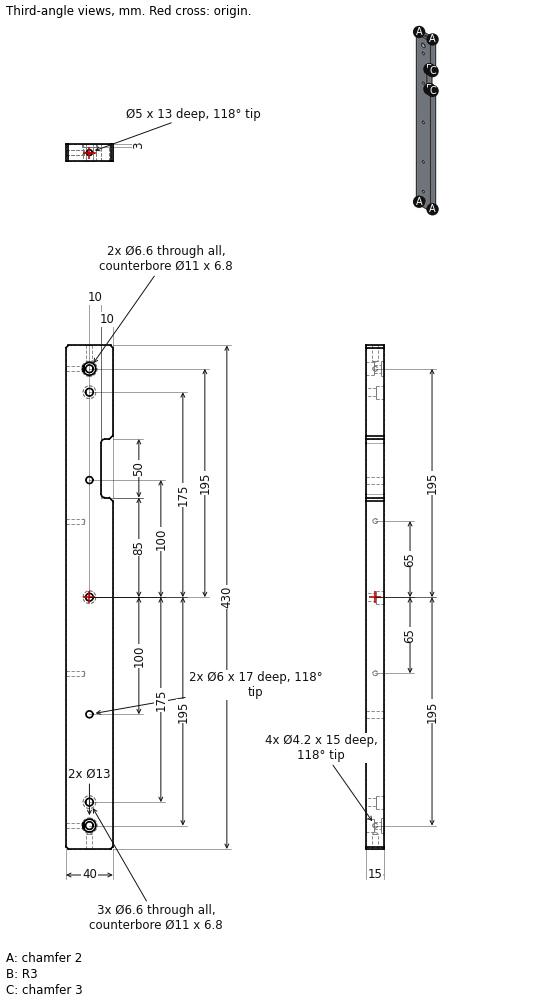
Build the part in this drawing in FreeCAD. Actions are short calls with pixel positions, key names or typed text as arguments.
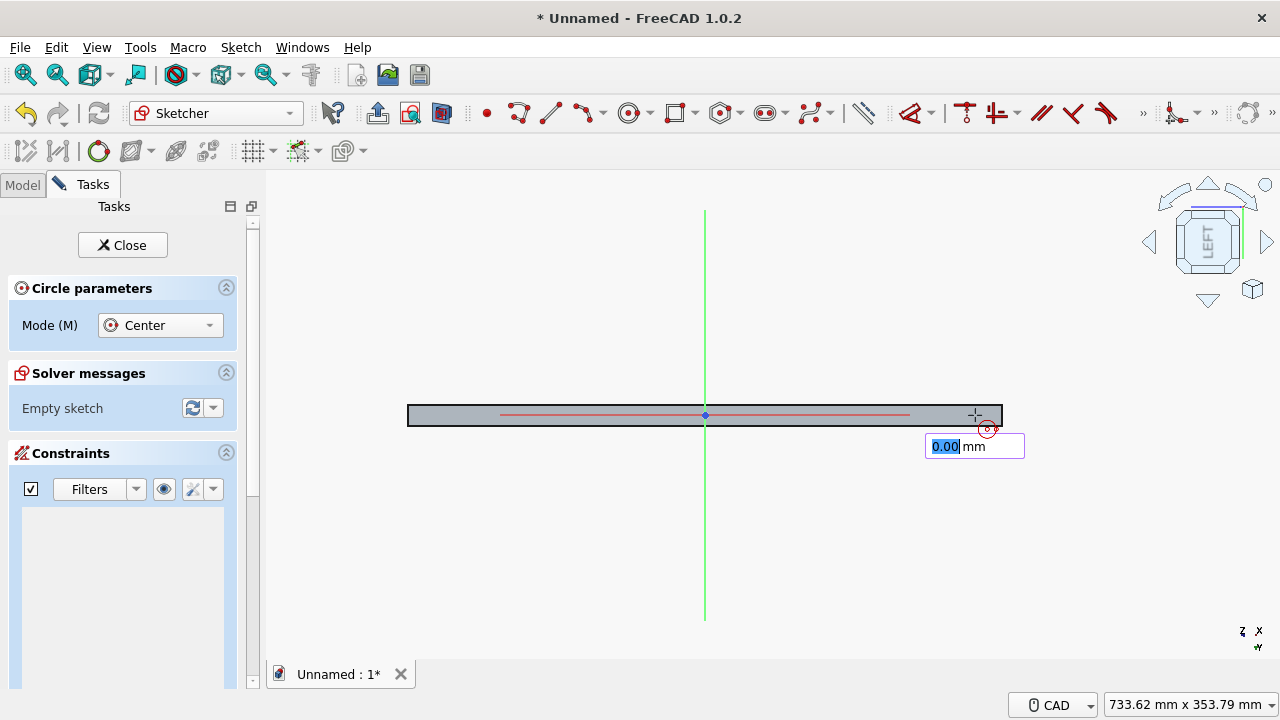
scroll(976, 412, up, 9)
move(971, 412)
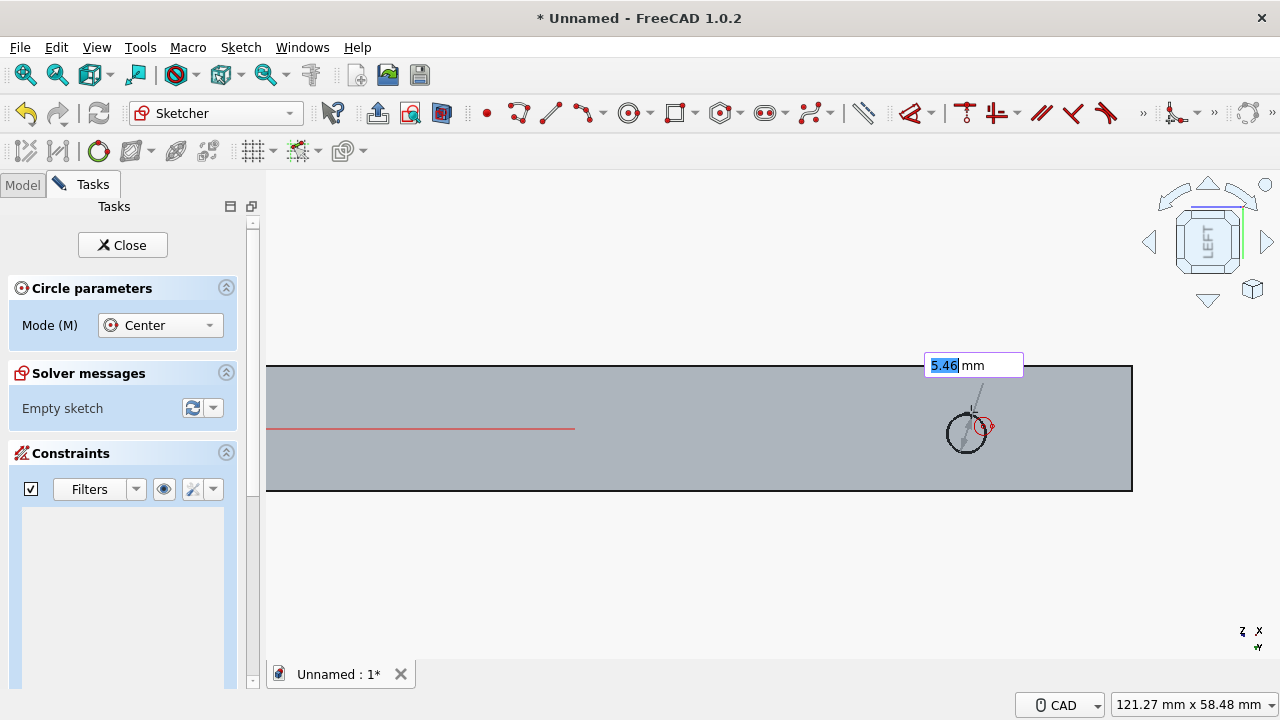
text(4.2)
key(Return)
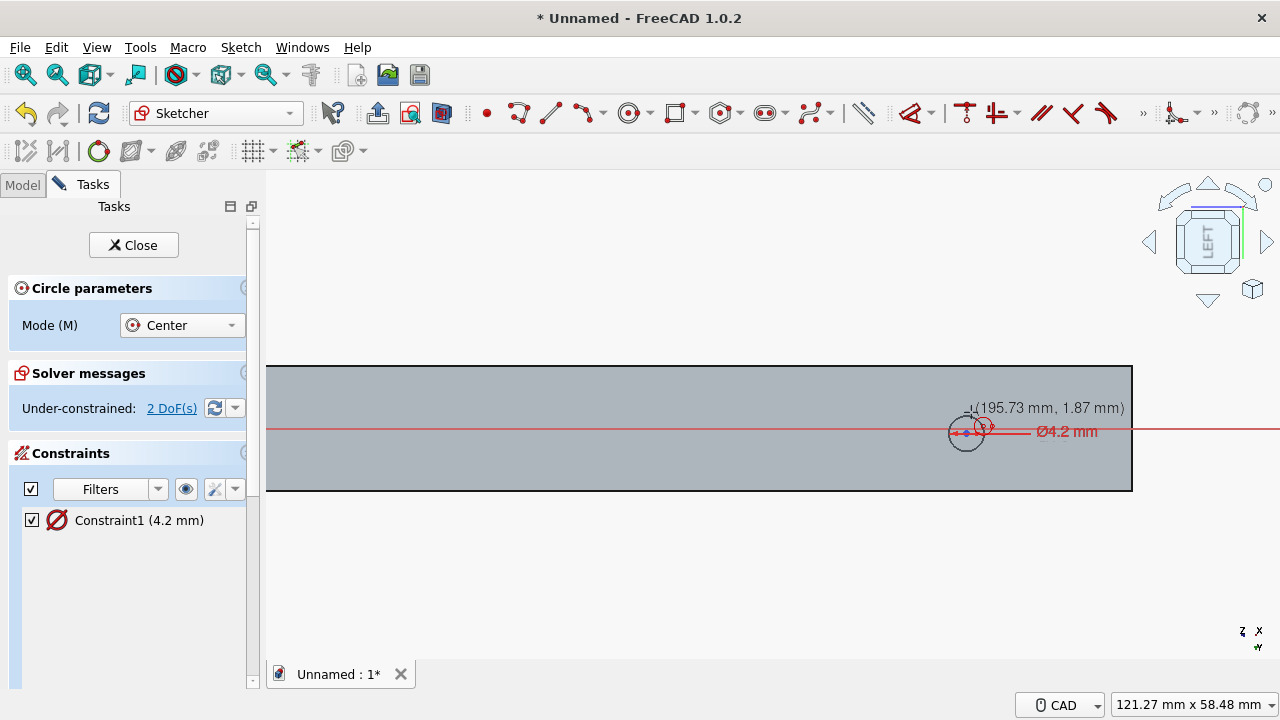
scroll(976, 412, down, 9)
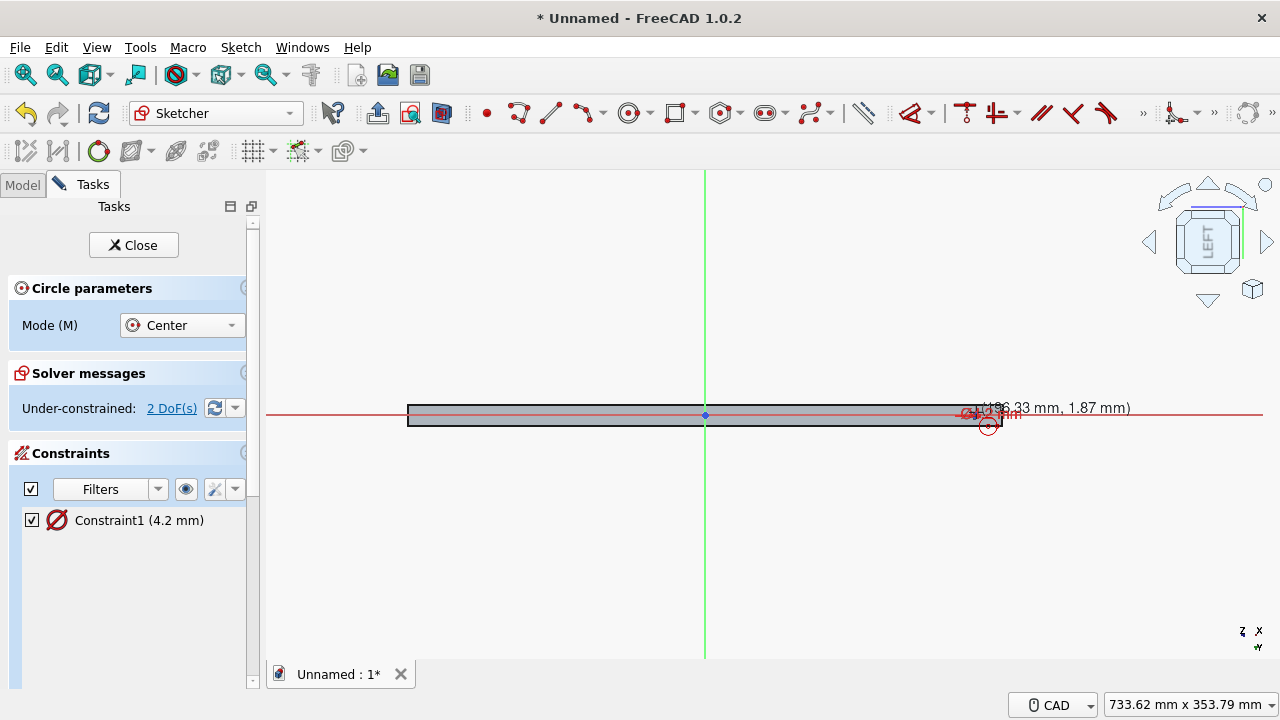
scroll(436, 415, up, 11)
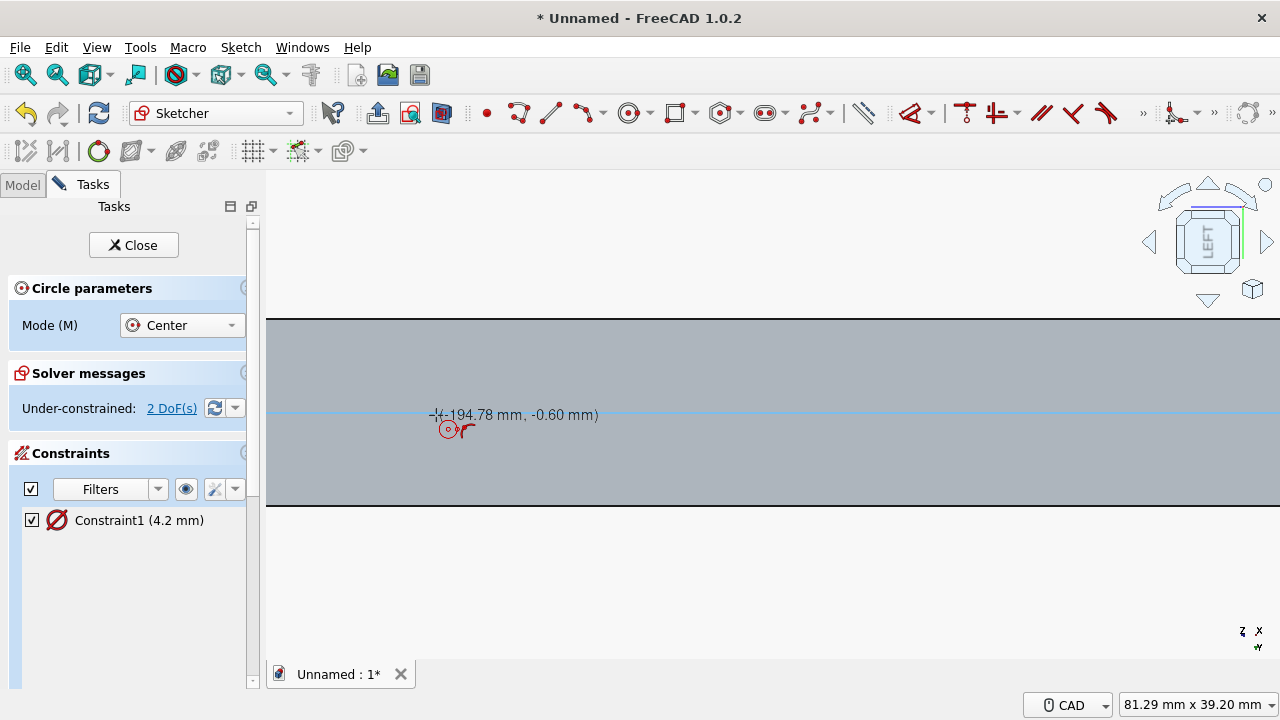
scroll(435, 415, down, 11)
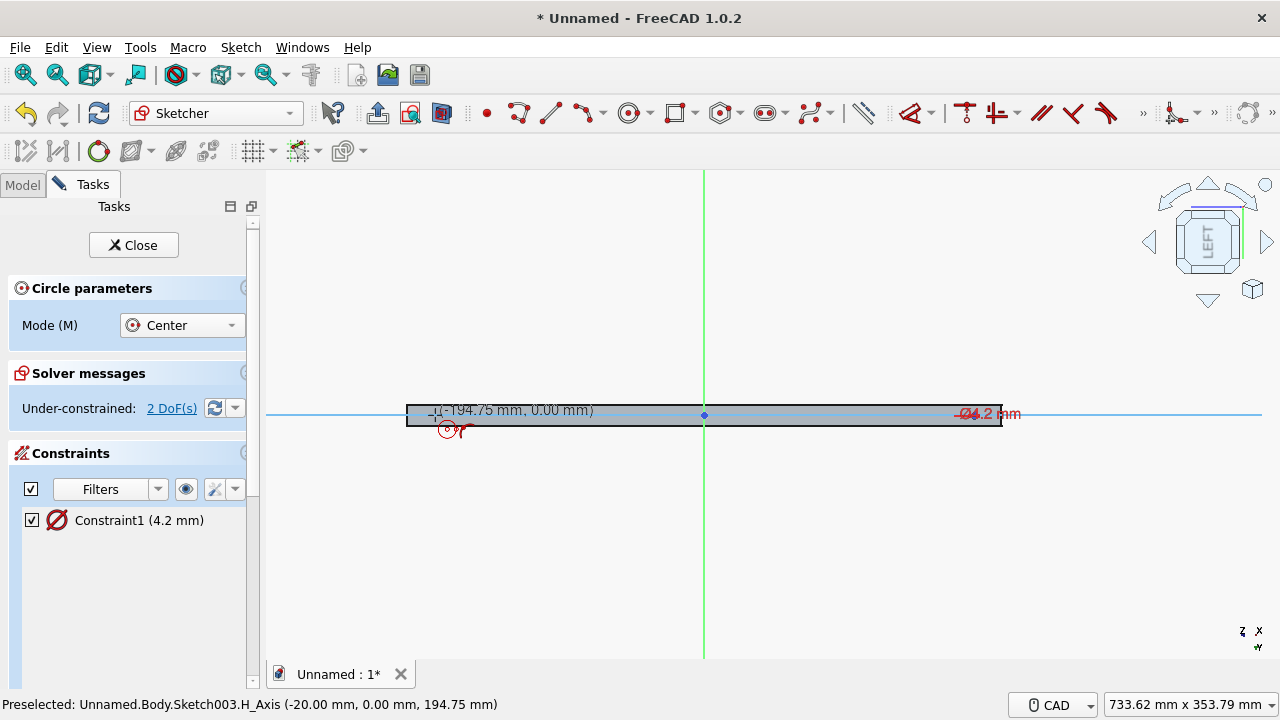
click(435, 415)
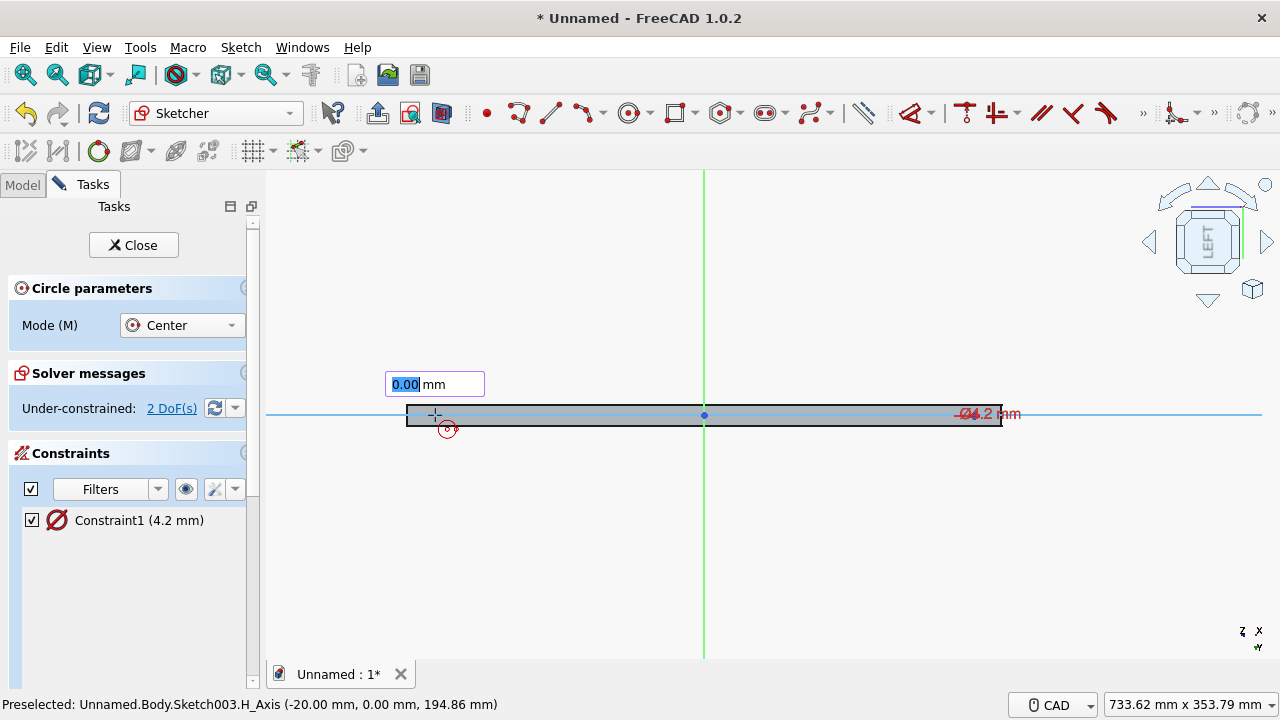
scroll(434, 418, up, 9)
move(432, 415)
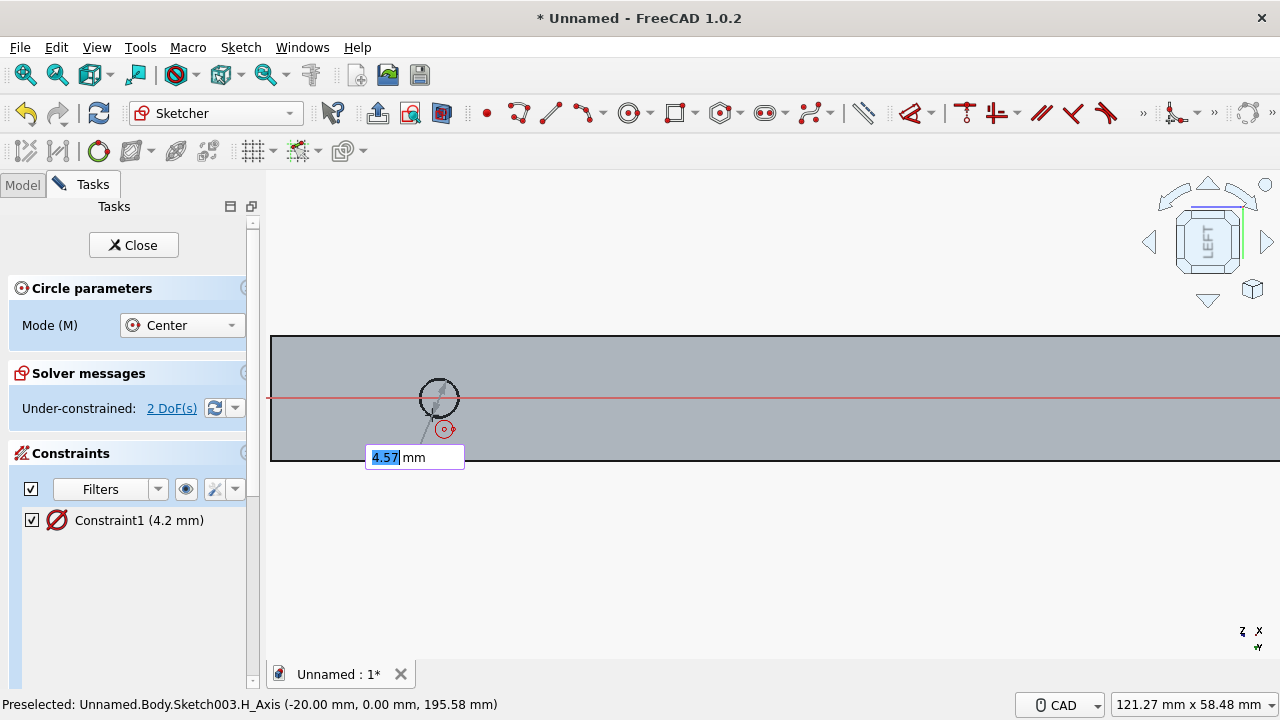
text(4.2)
key(Return)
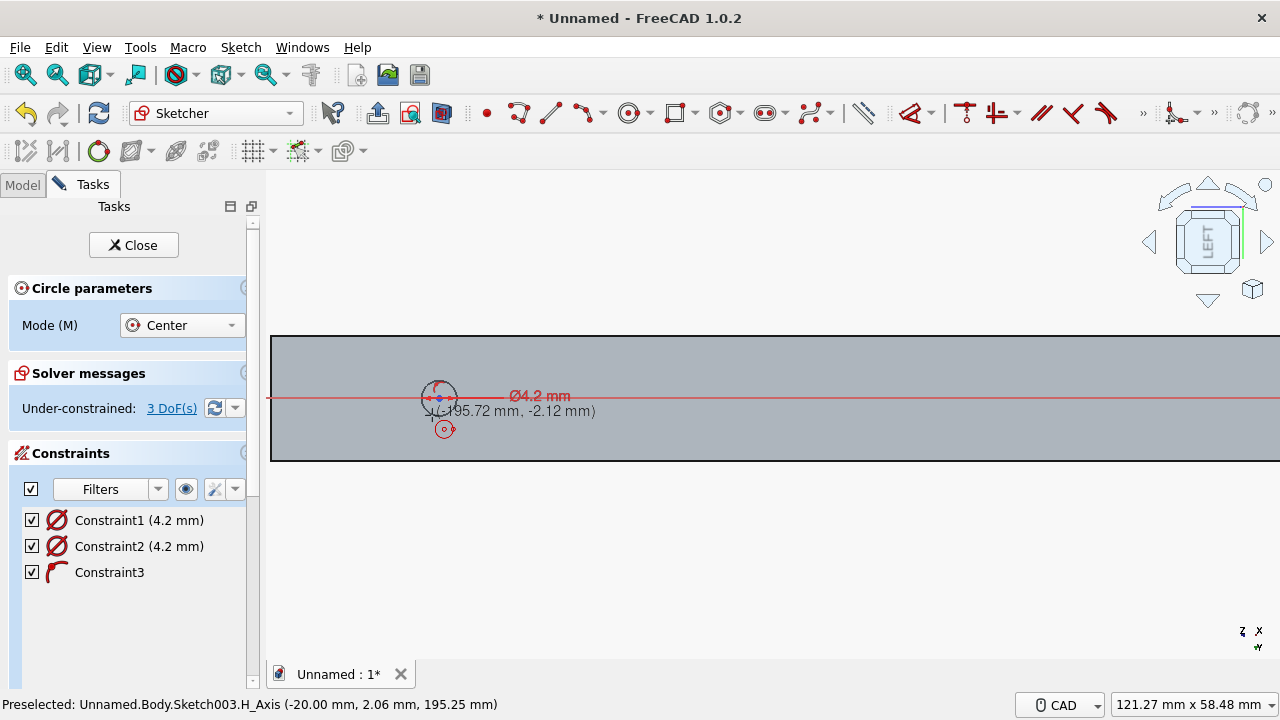
scroll(434, 418, down, 9)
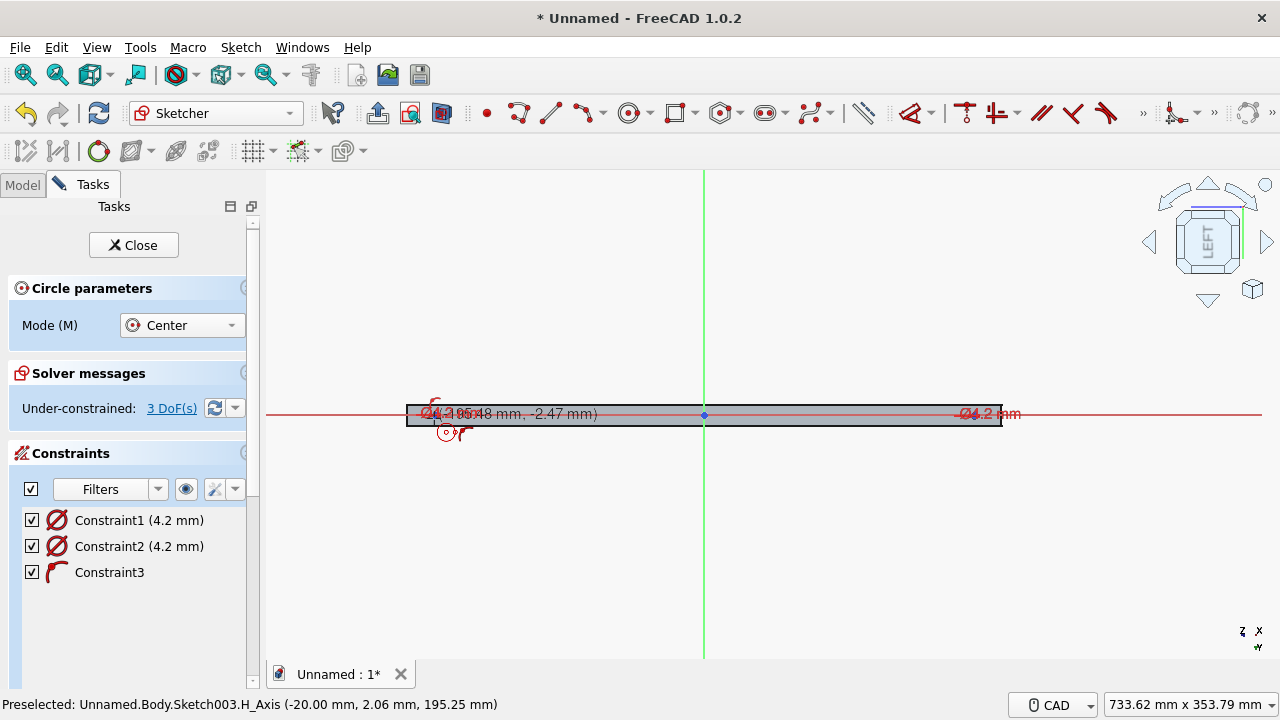
scroll(794, 415, up, 11)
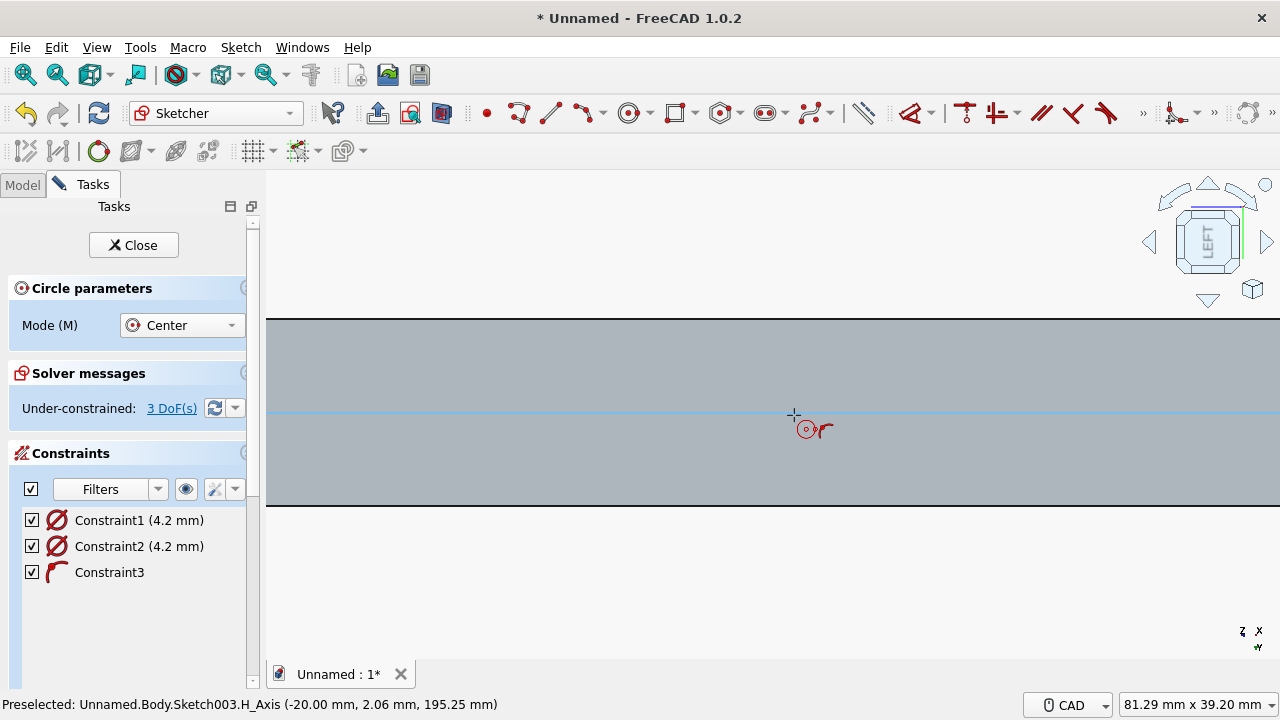
scroll(795, 415, down, 11)